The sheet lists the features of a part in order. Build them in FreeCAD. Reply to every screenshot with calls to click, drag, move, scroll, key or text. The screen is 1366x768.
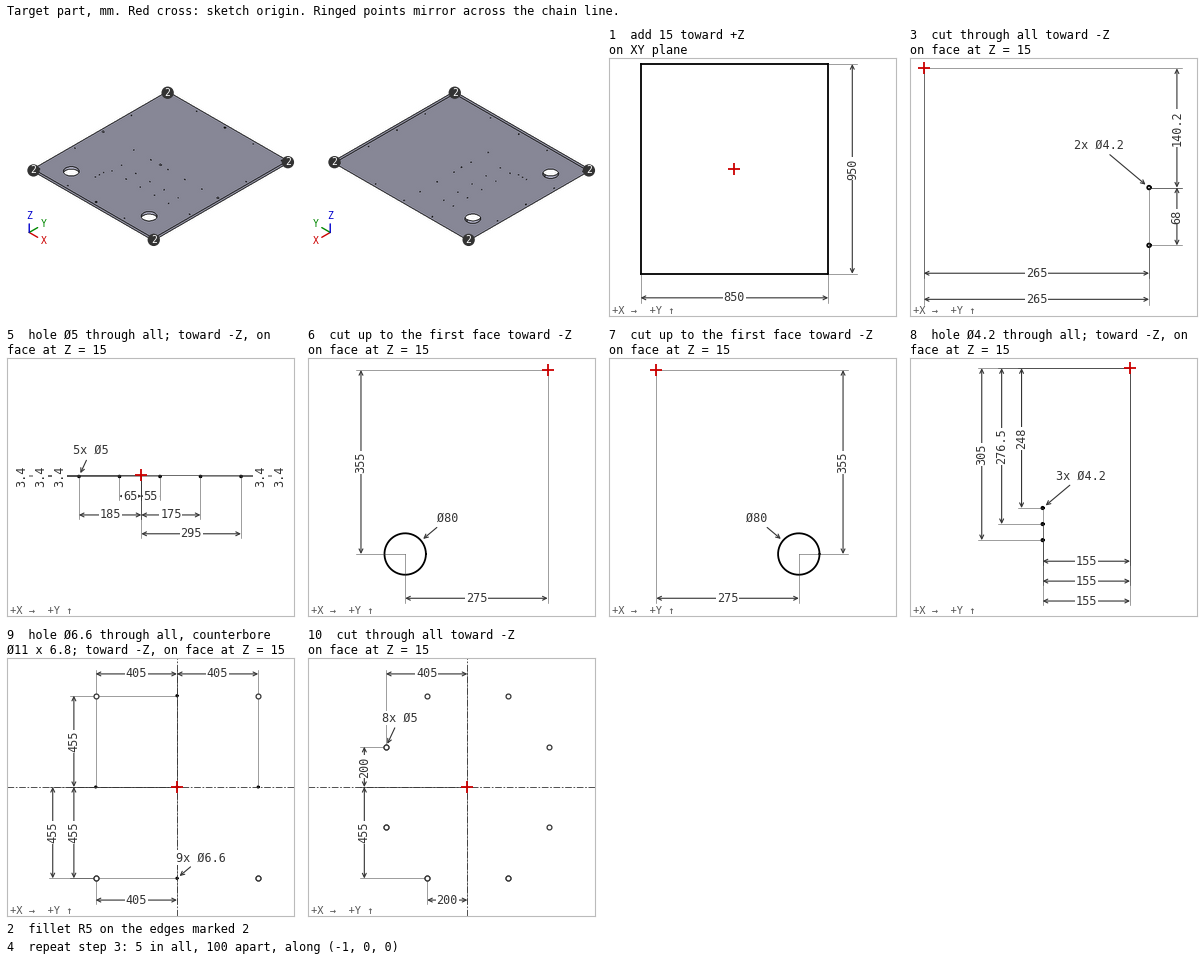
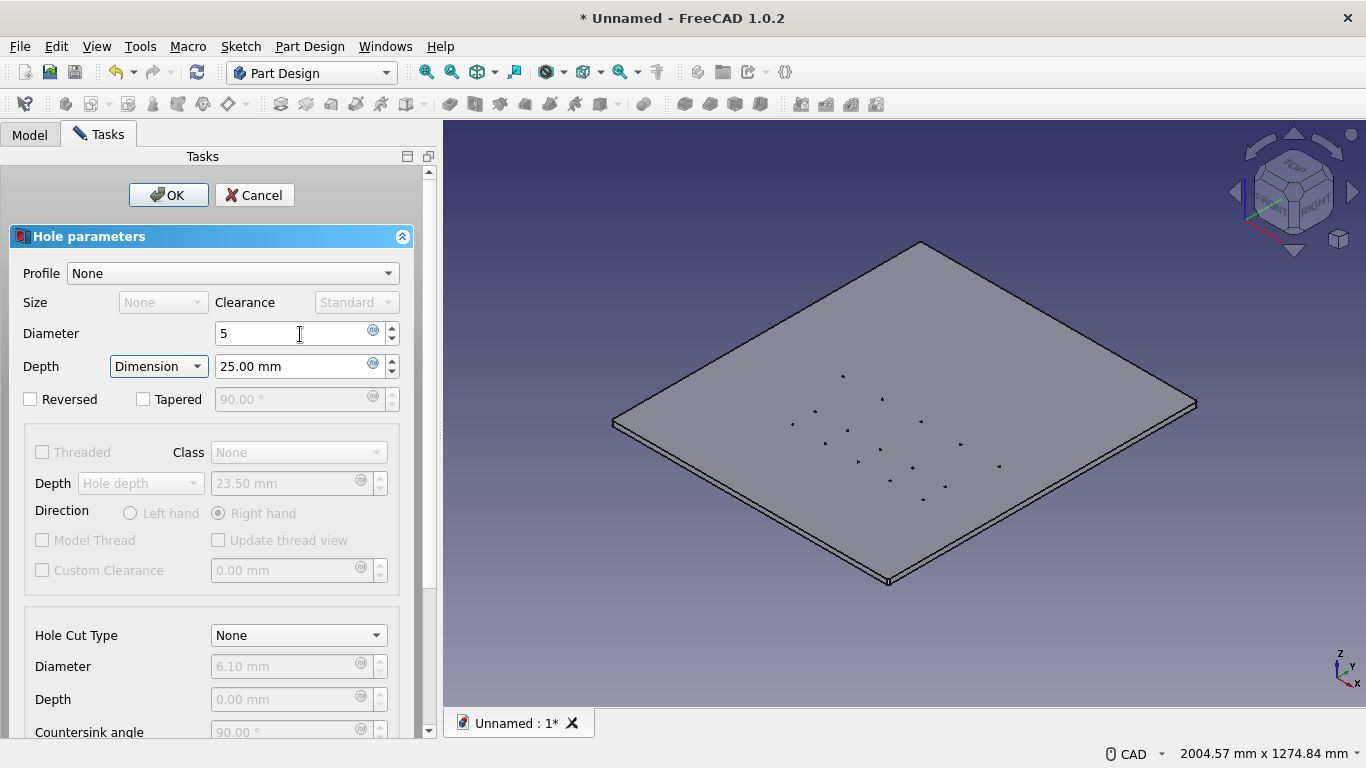
click(160, 366)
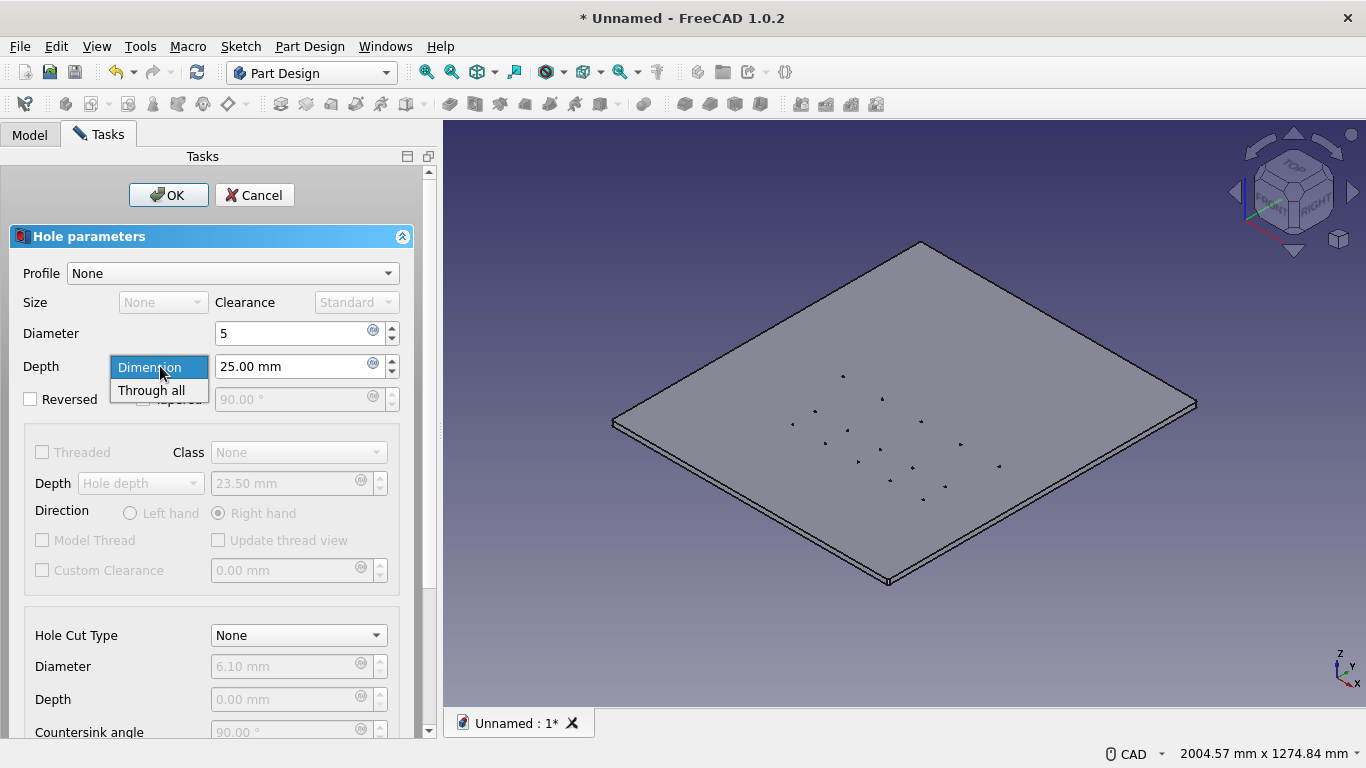
click(158, 390)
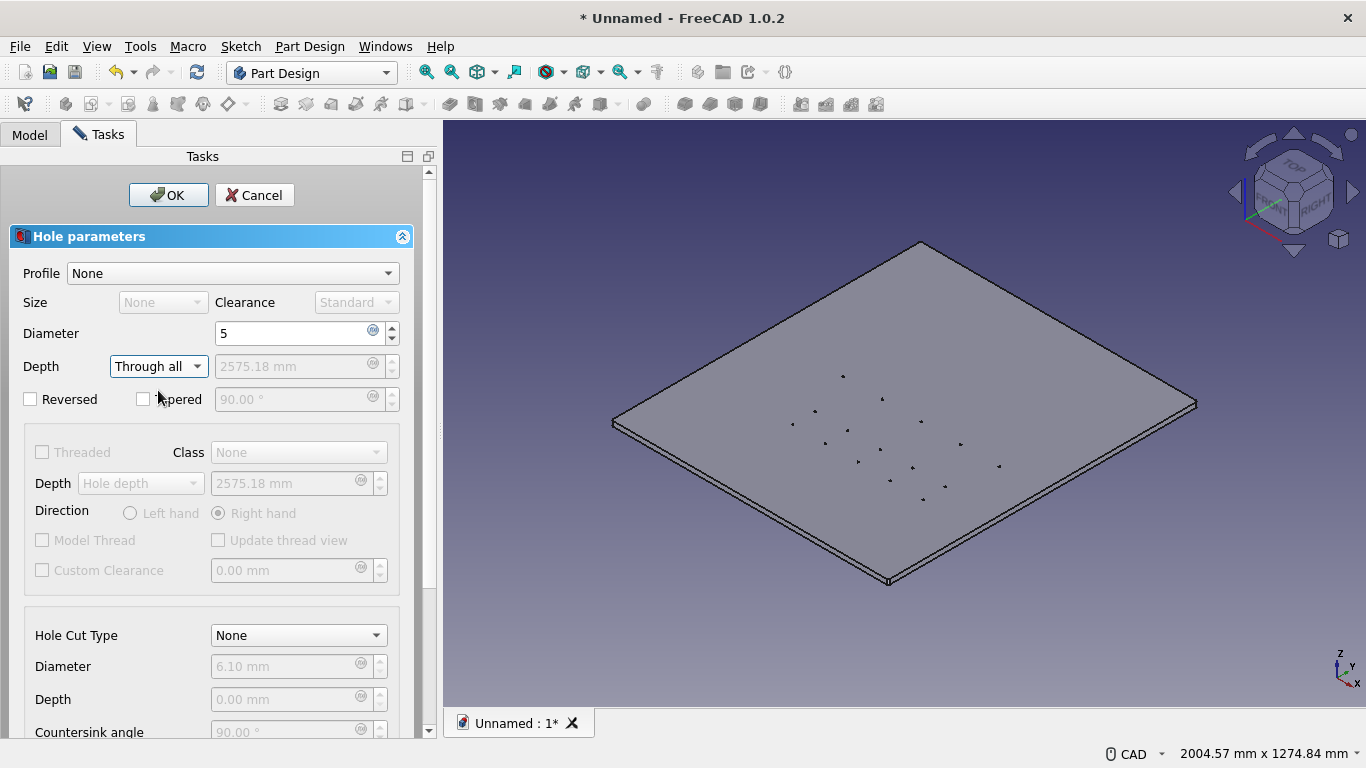
click(169, 195)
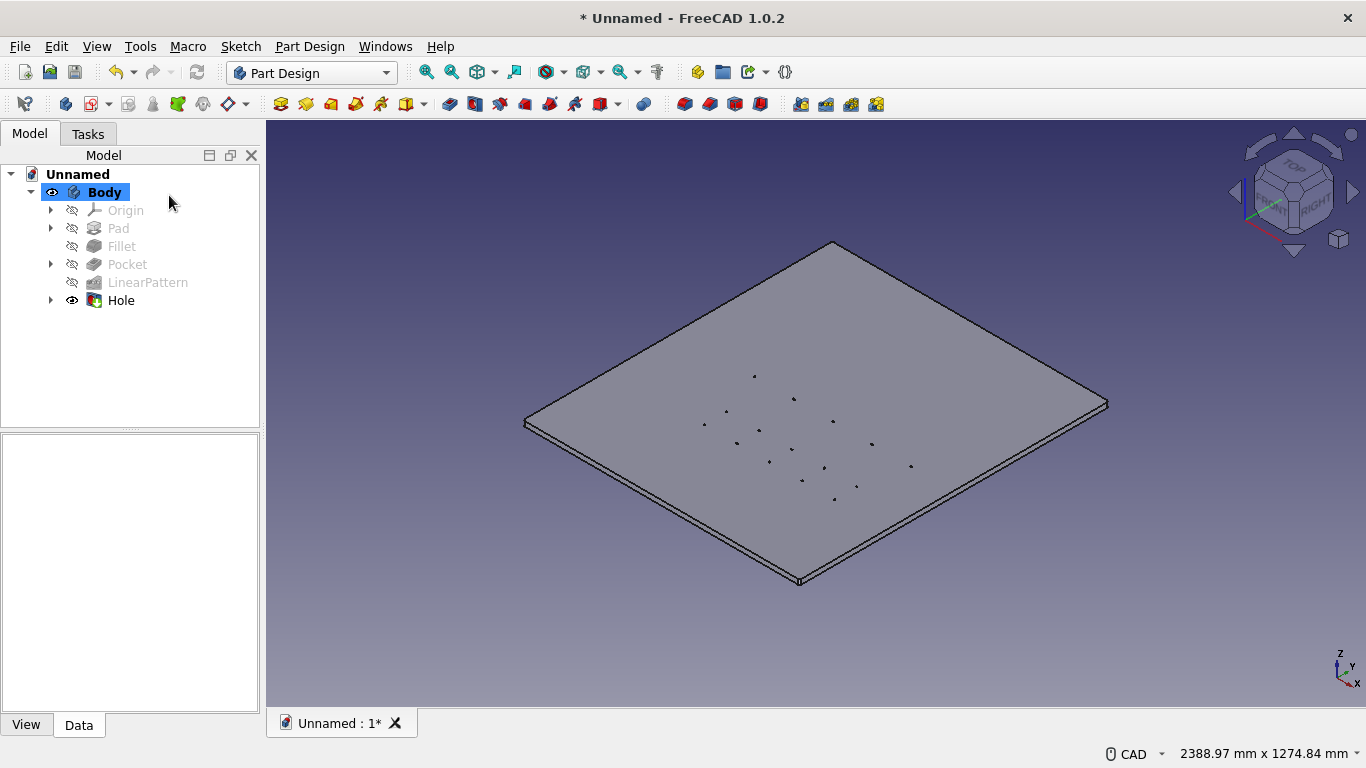
click(944, 381)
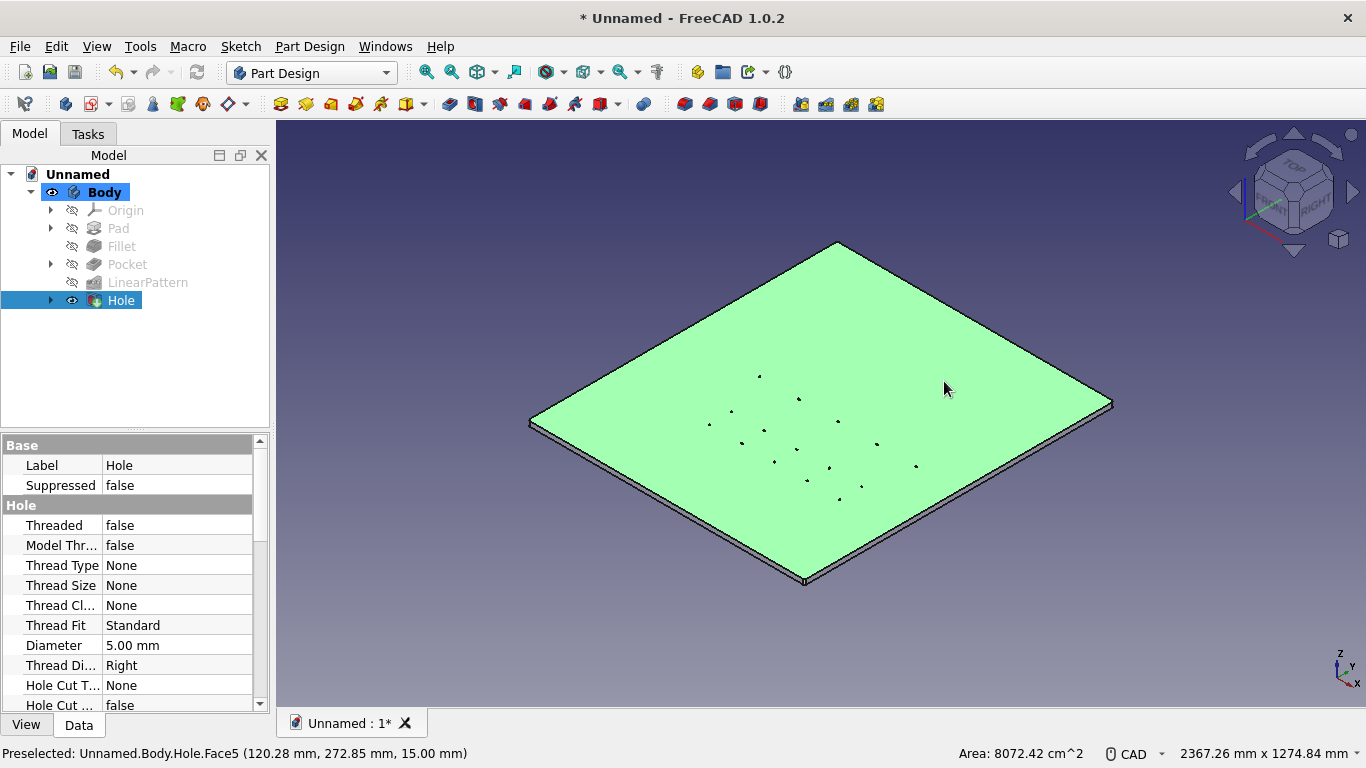
click(90, 104)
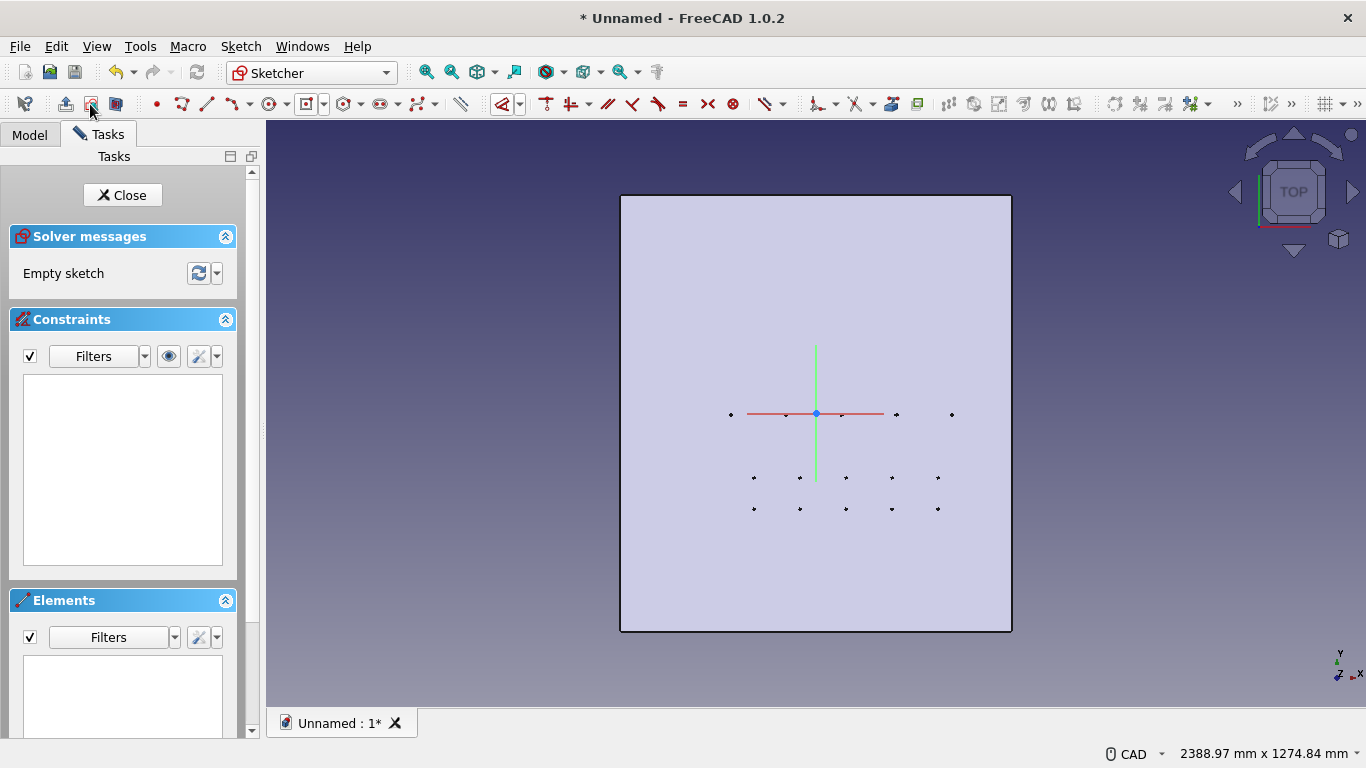
scroll(684, 593, up, 12)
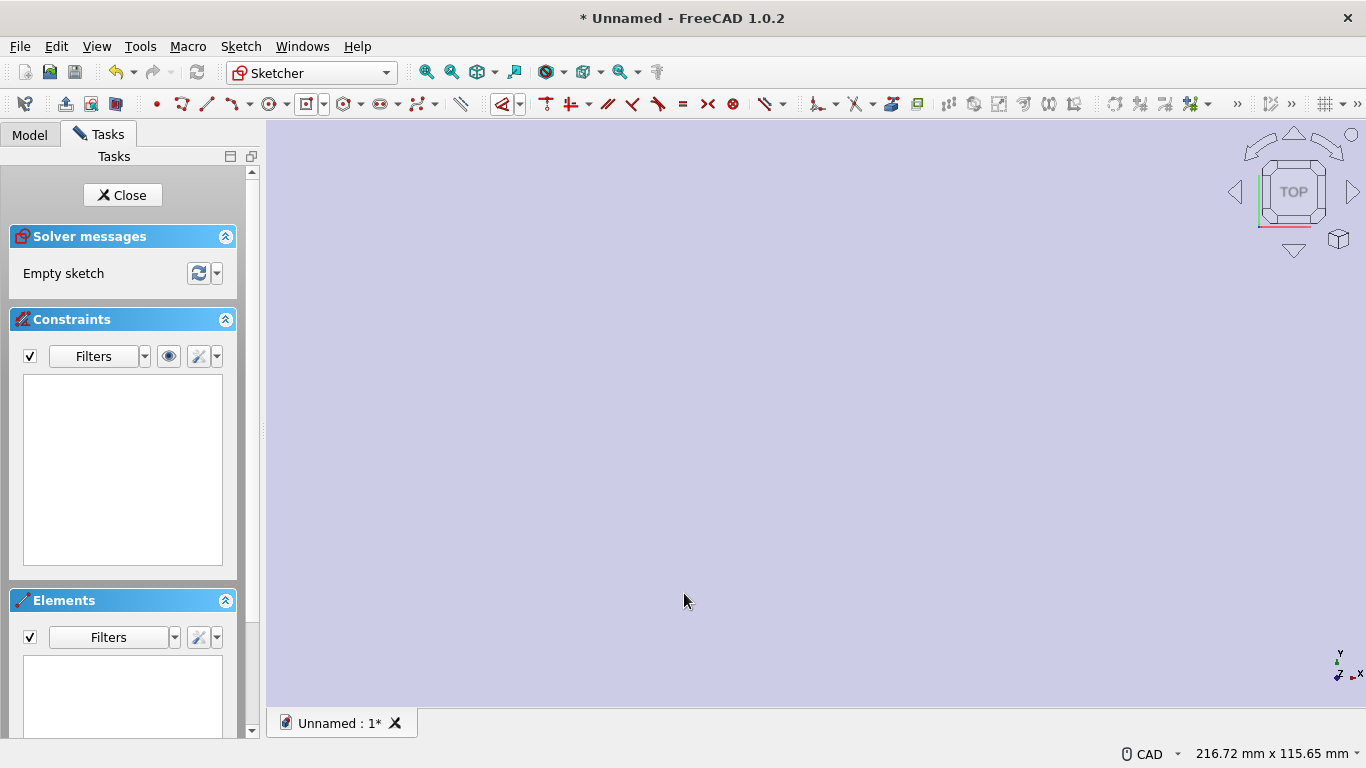
click(268, 104)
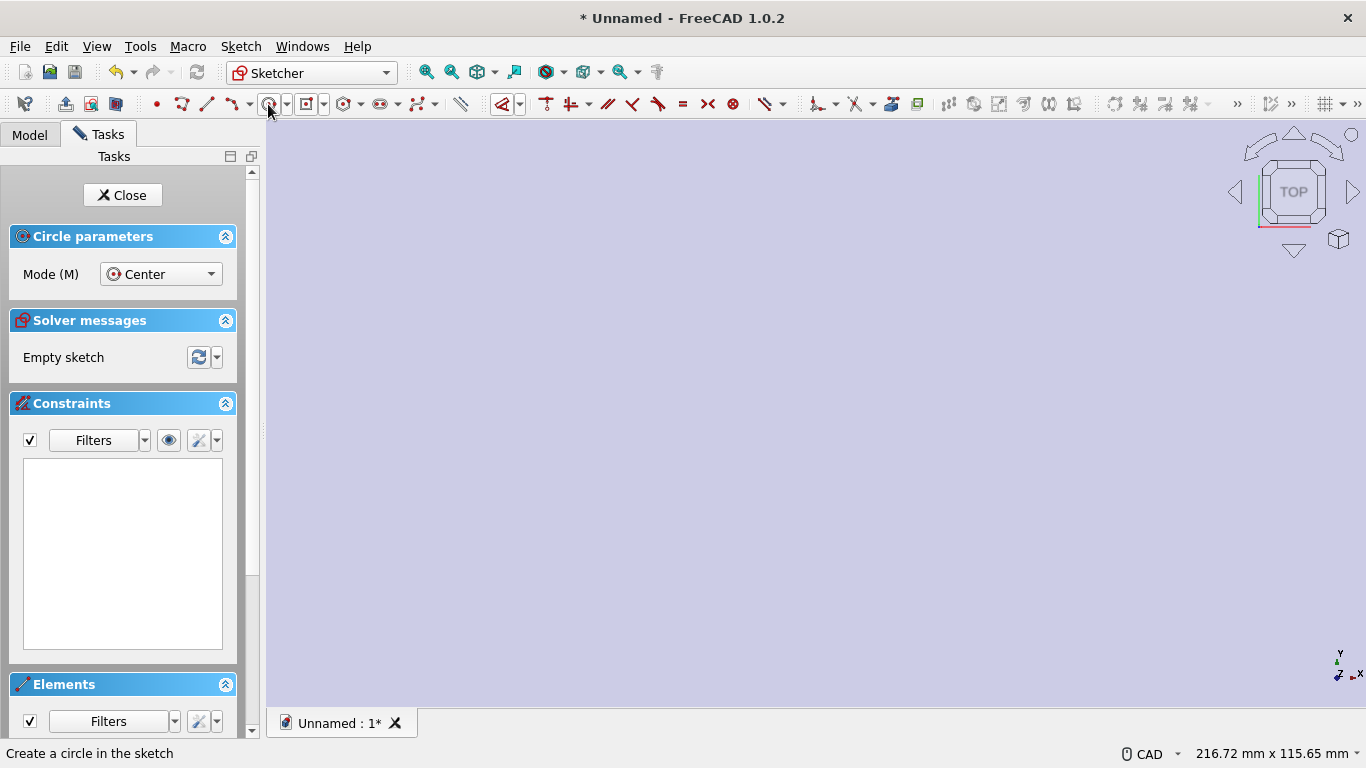
click(739, 408)
move(883, 265)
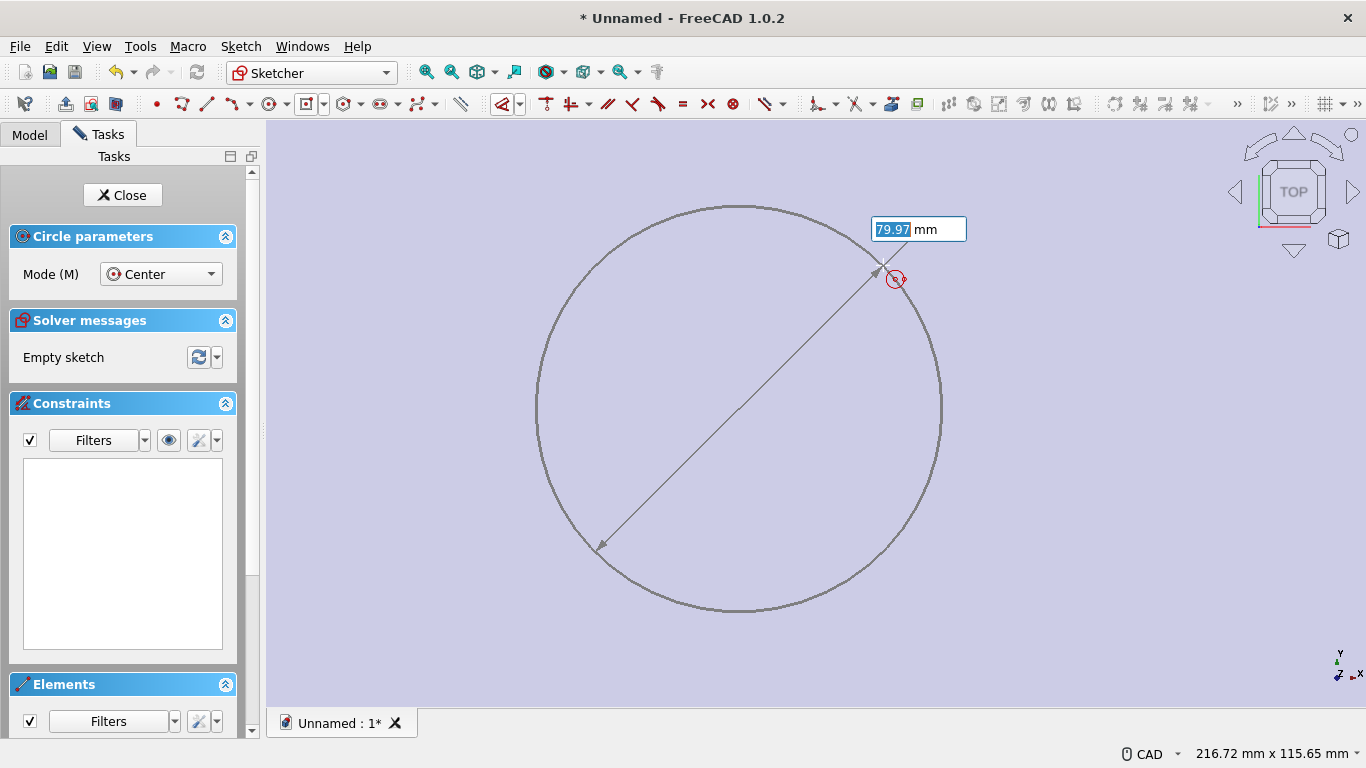
text(80)
key(Return)
key(Escape)